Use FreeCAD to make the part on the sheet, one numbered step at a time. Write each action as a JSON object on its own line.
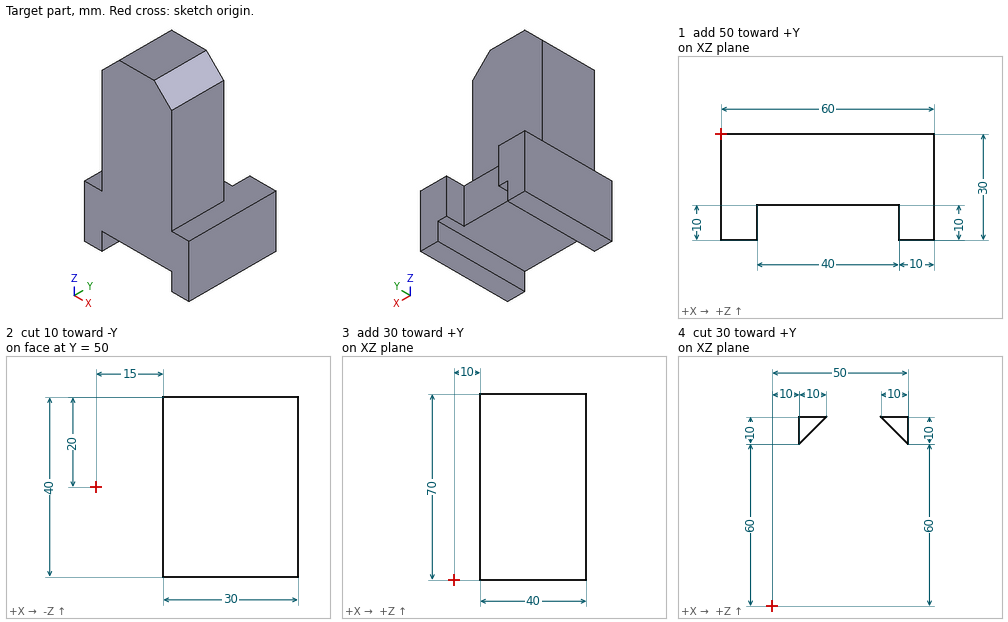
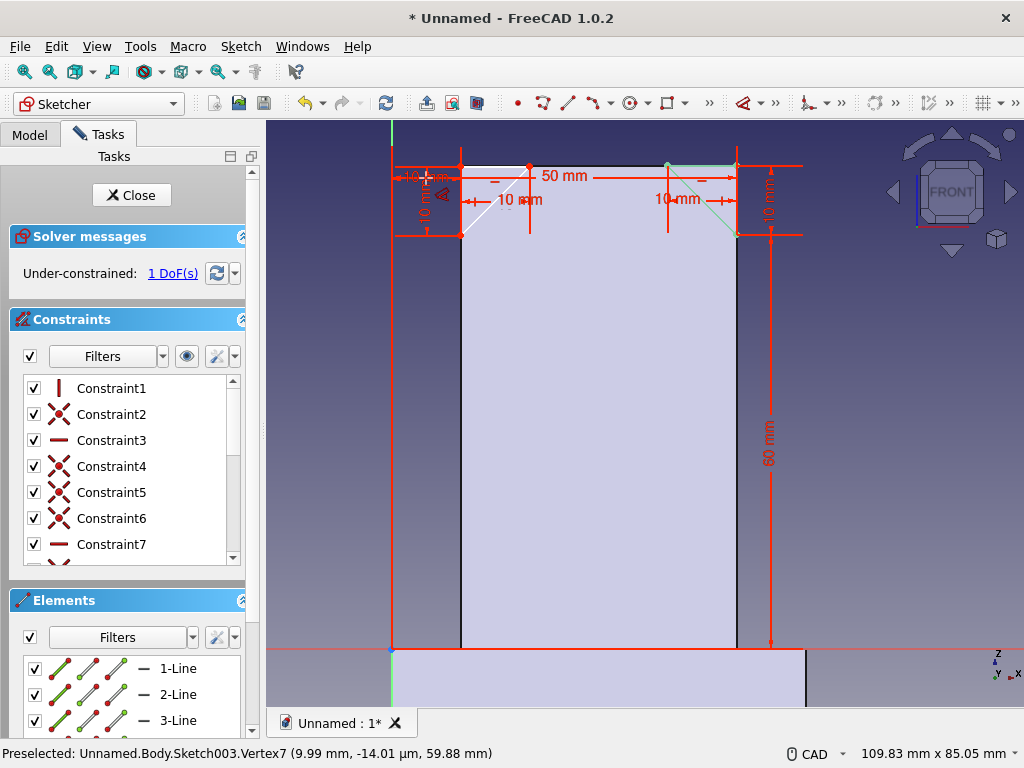
{"action": "left_click", "coordinate": [461, 236]}
{"action": "left_click", "coordinate": [358, 442]}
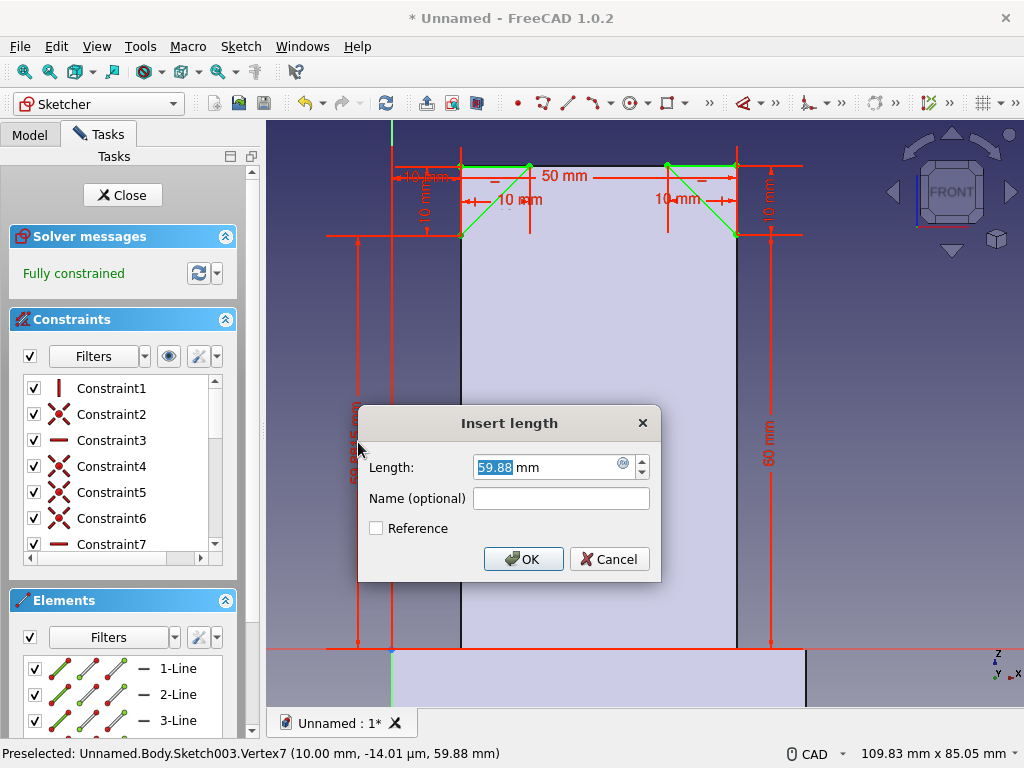
{"action": "type", "text": "60"}
{"action": "key", "text": "Return"}
{"action": "key", "text": "Escape"}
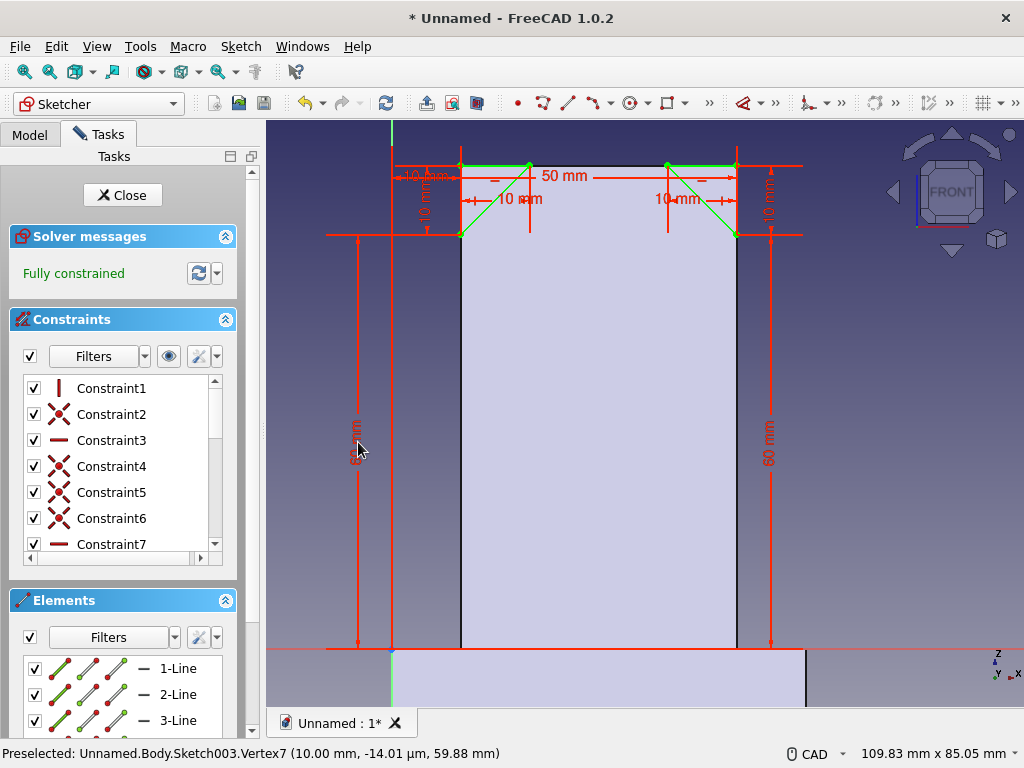
{"action": "left_click", "coordinate": [123, 195]}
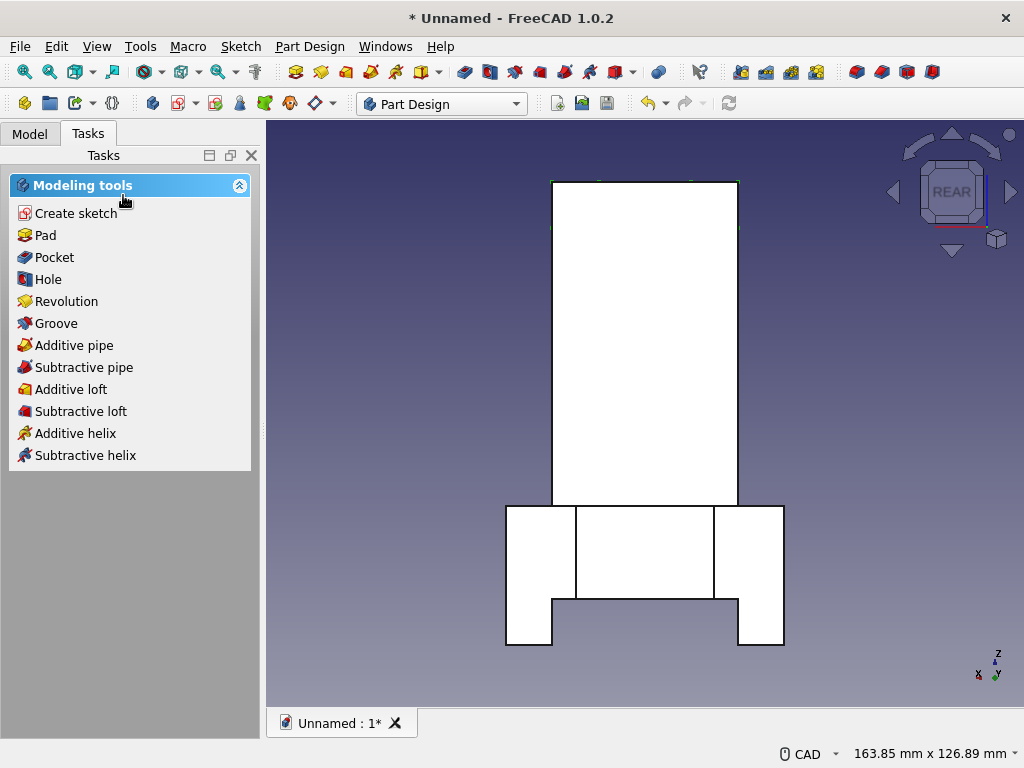
{"action": "left_click", "coordinate": [465, 72]}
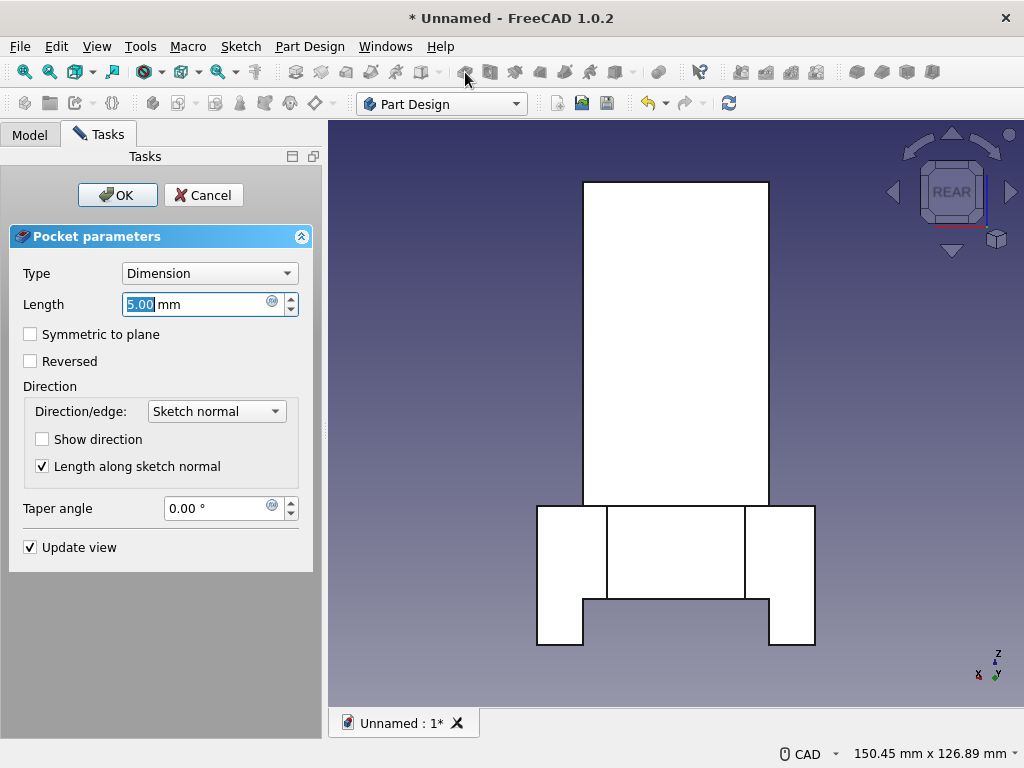
{"action": "type", "text": "30"}
{"action": "key", "text": "Tab"}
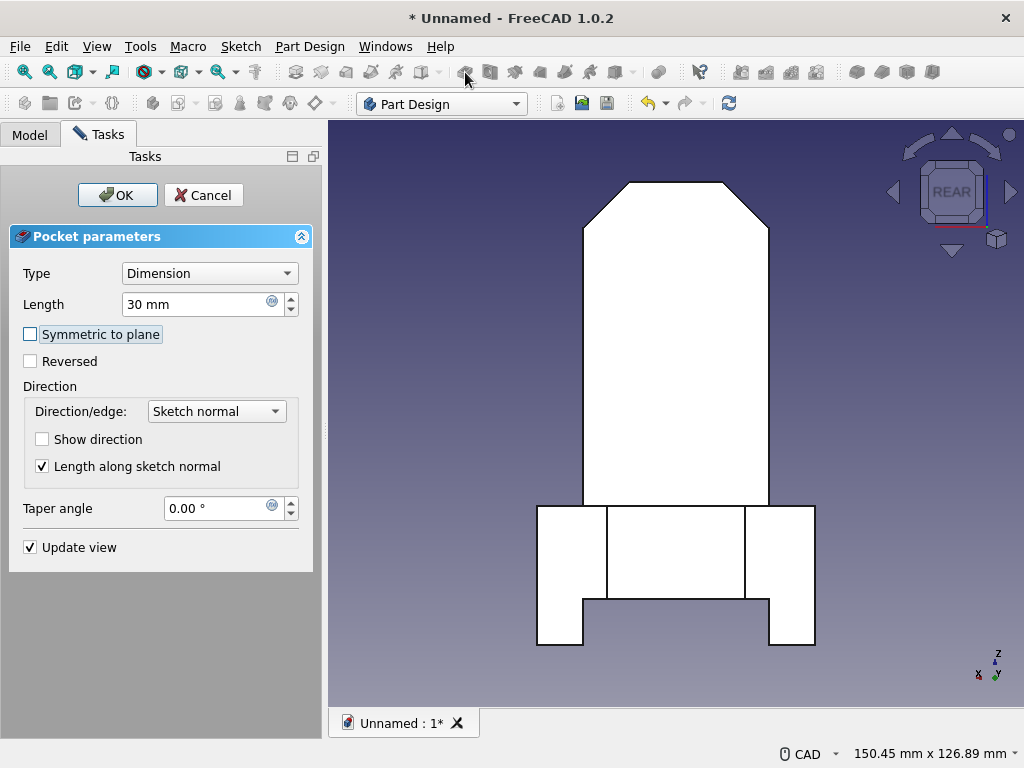
{"action": "left_click", "coordinate": [118, 195]}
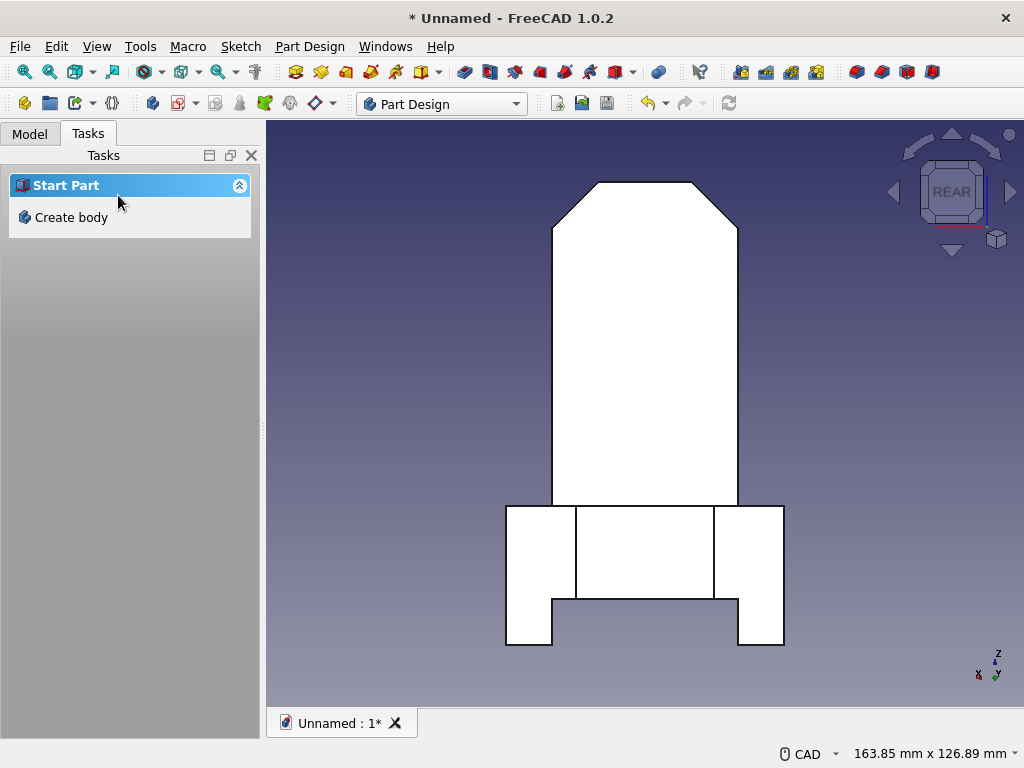
{"action": "key", "text": "0"}